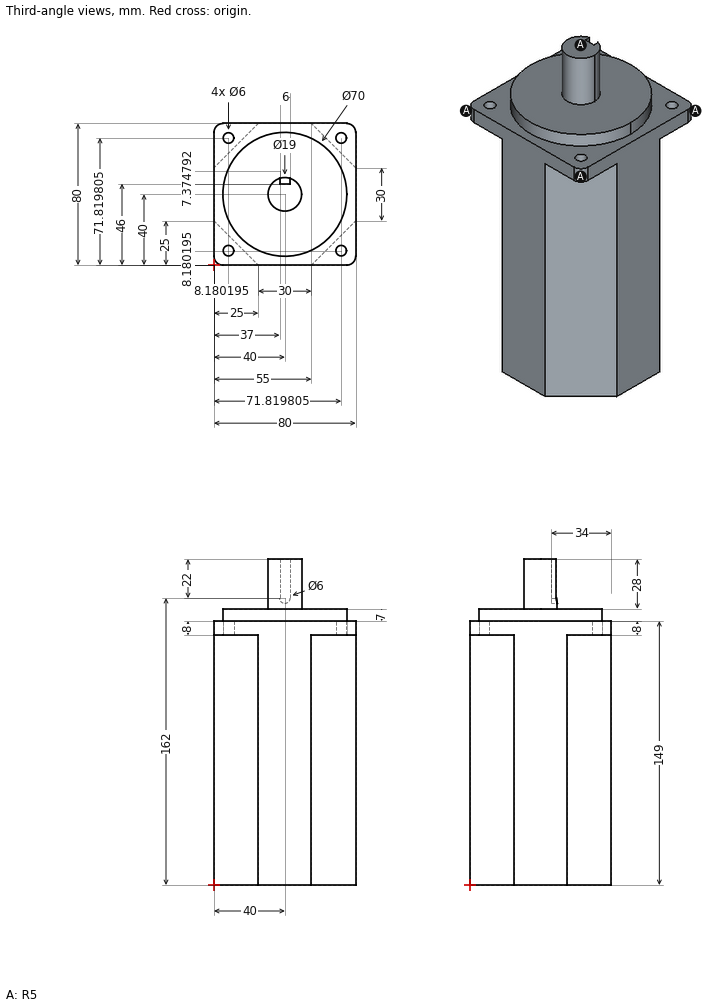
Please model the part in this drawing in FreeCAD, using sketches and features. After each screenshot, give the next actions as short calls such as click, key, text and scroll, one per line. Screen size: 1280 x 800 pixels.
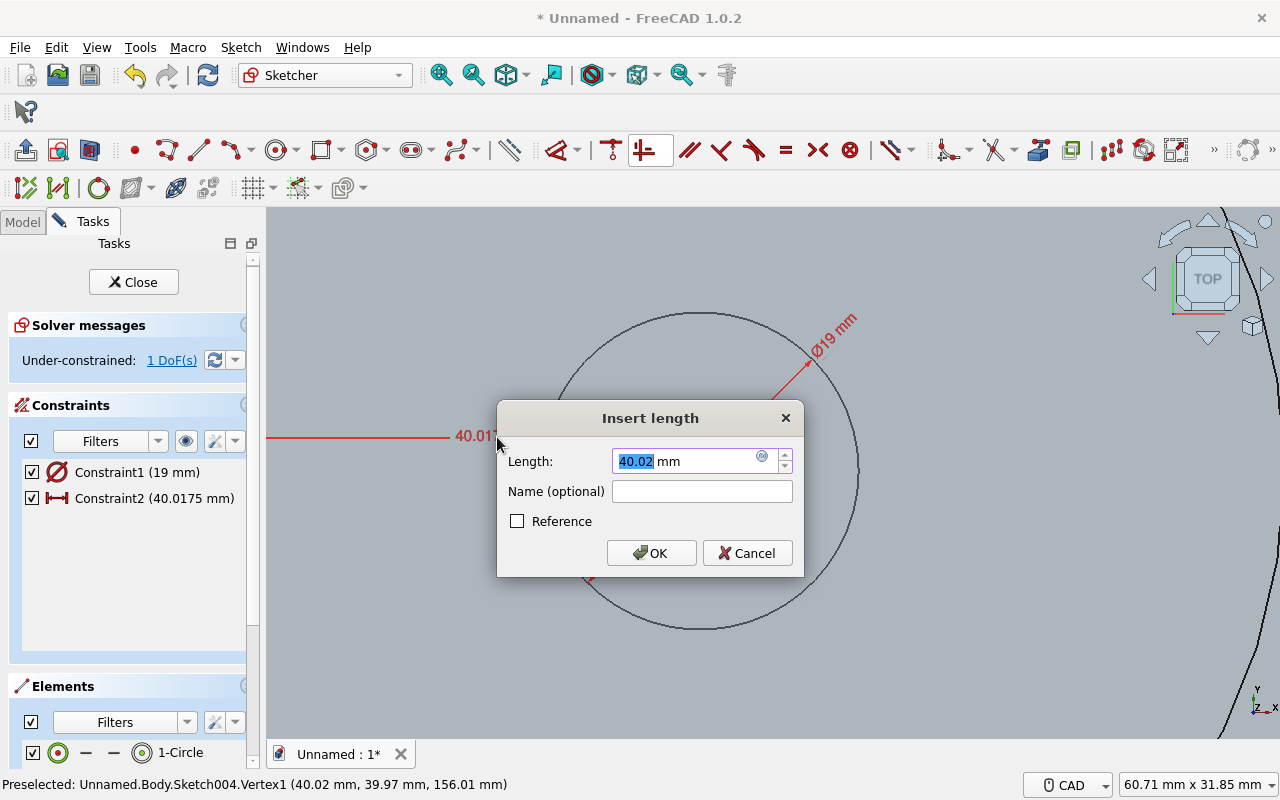
text(40)
key(Return)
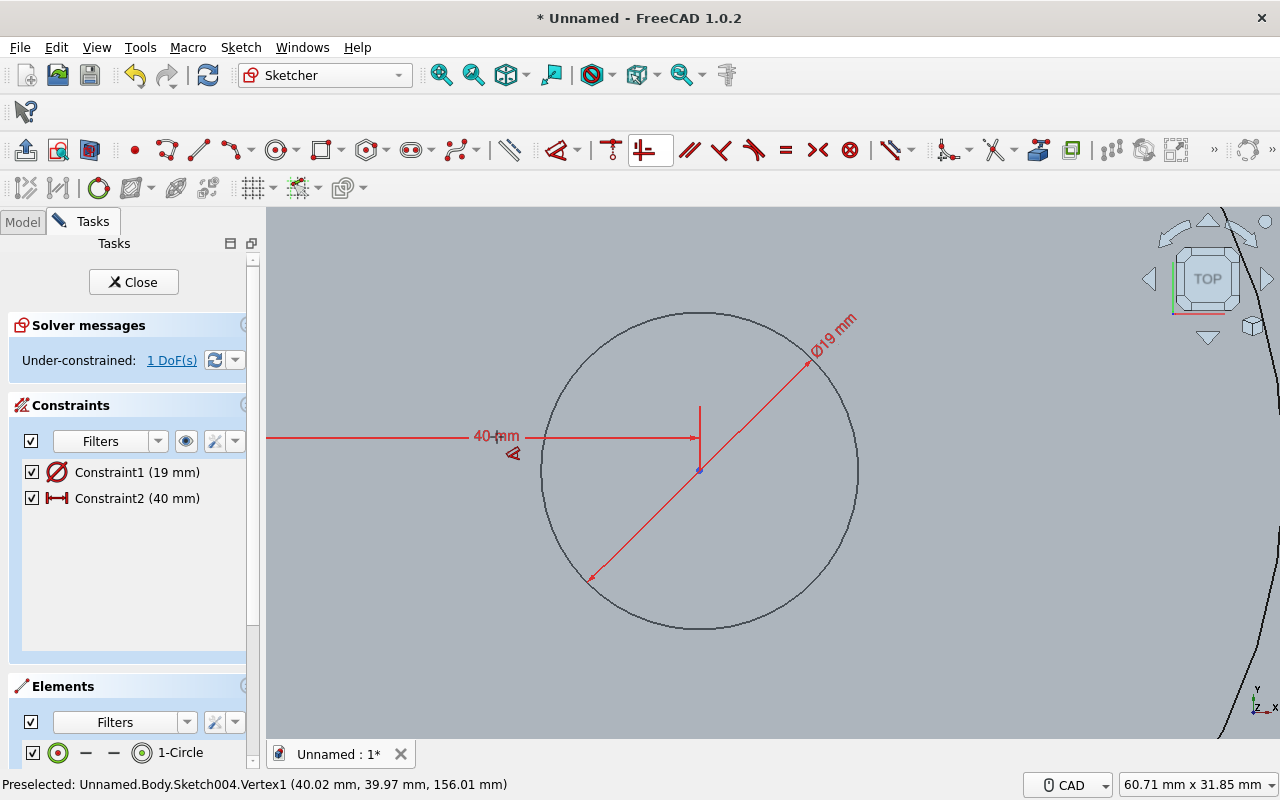
click(700, 471)
click(734, 591)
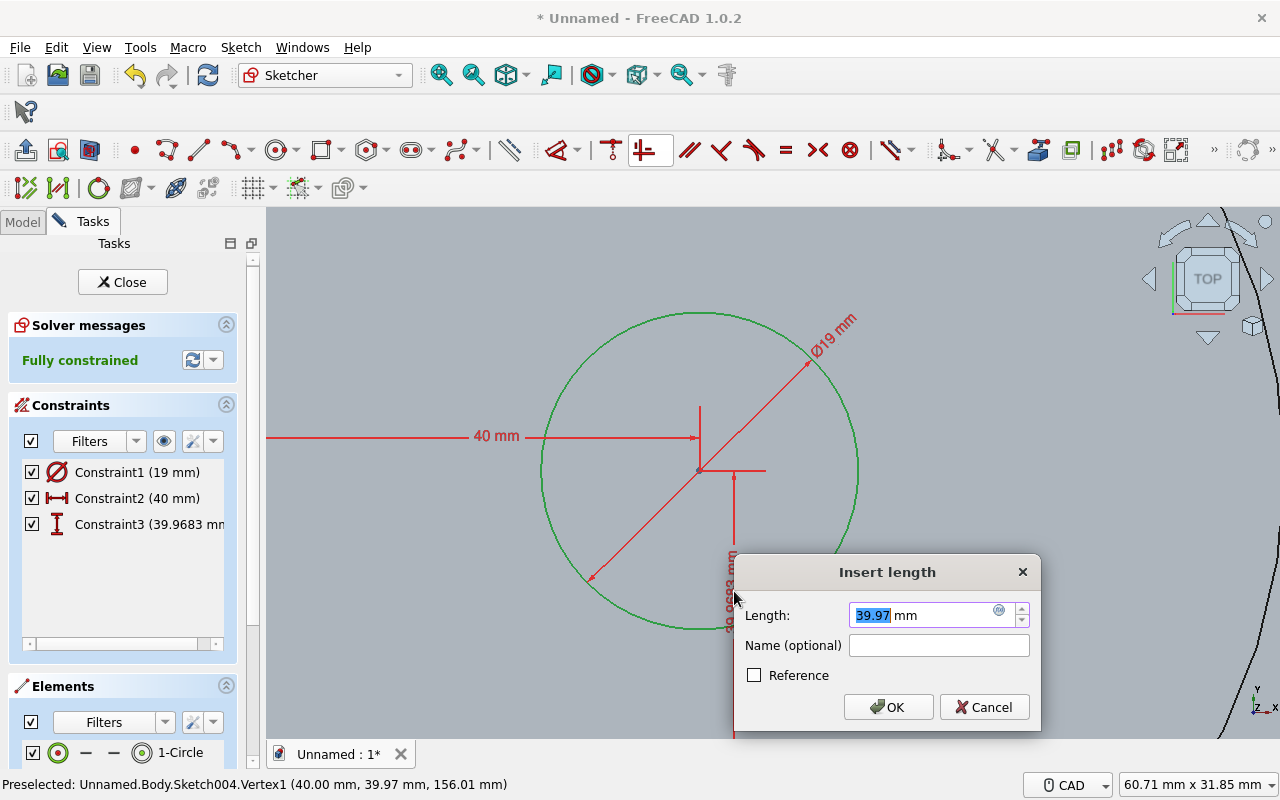
text(40)
key(Return)
key(Escape)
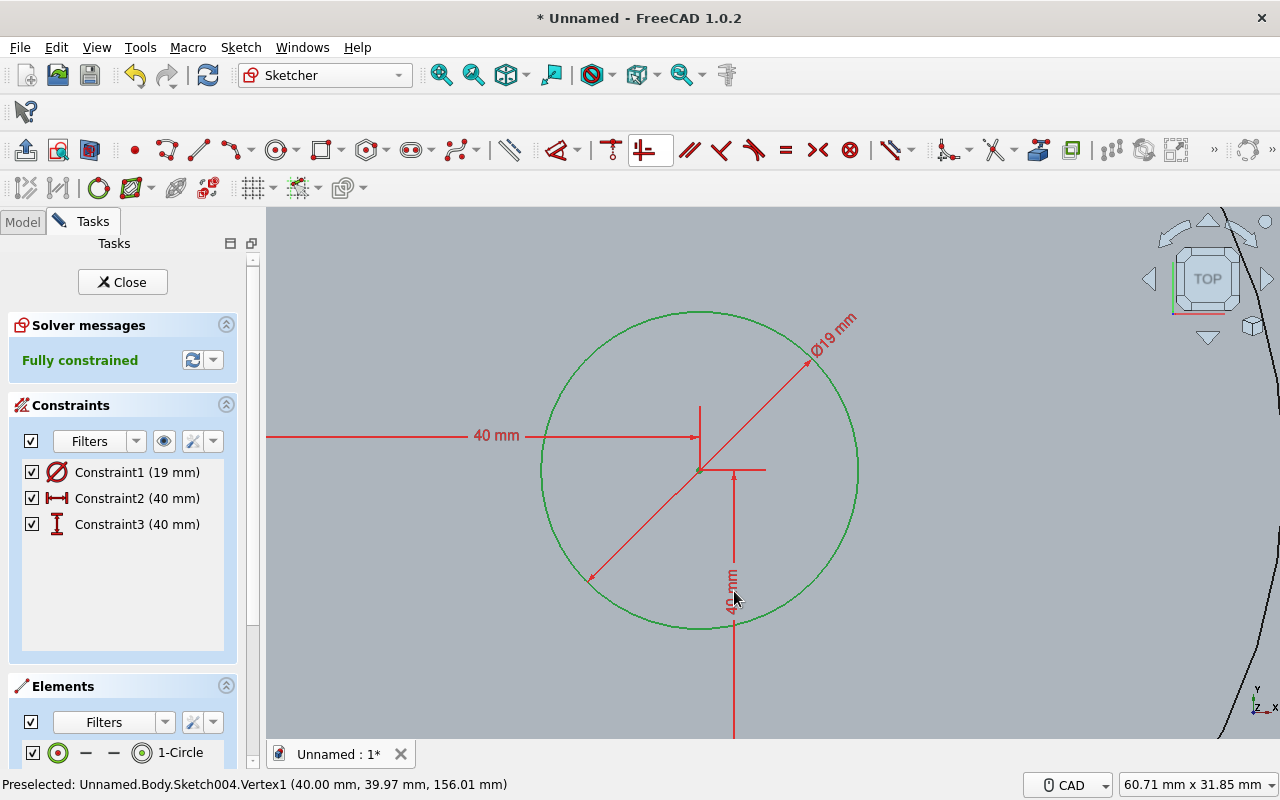
click(123, 282)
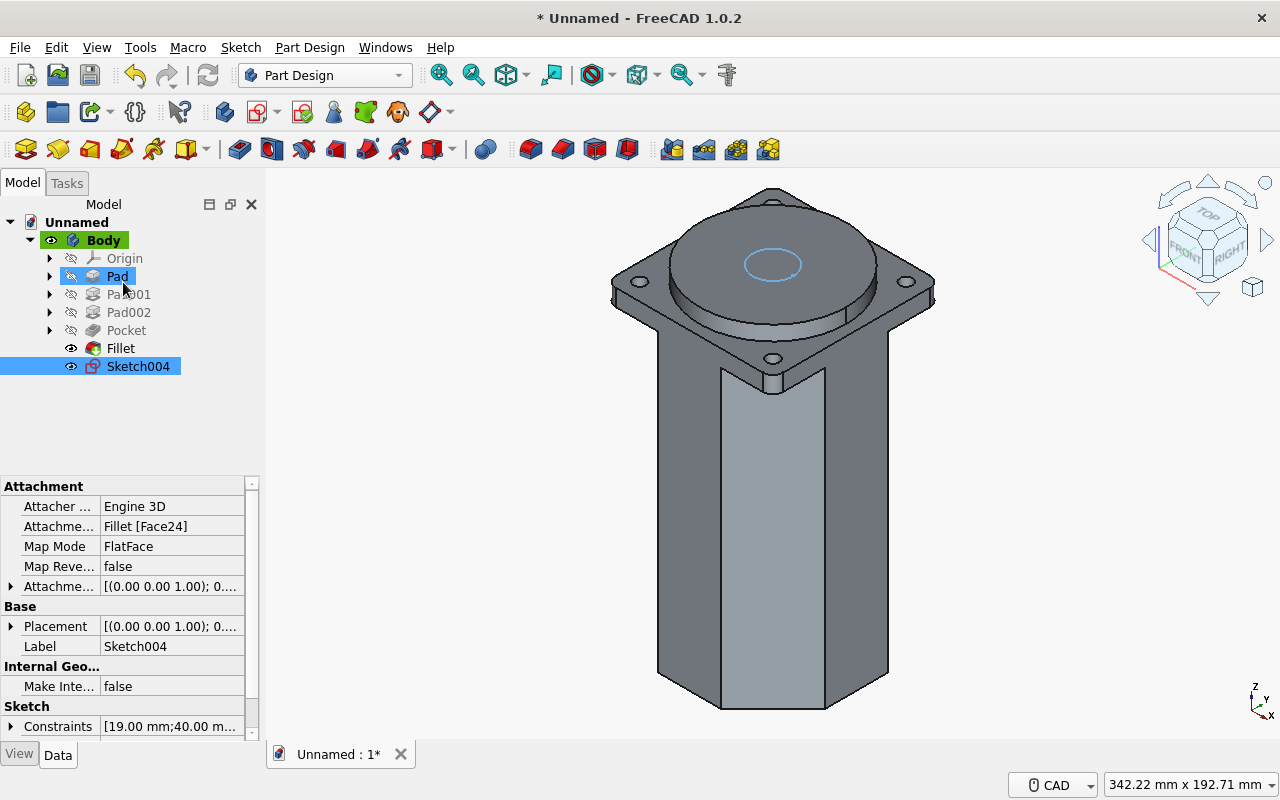
click(26, 150)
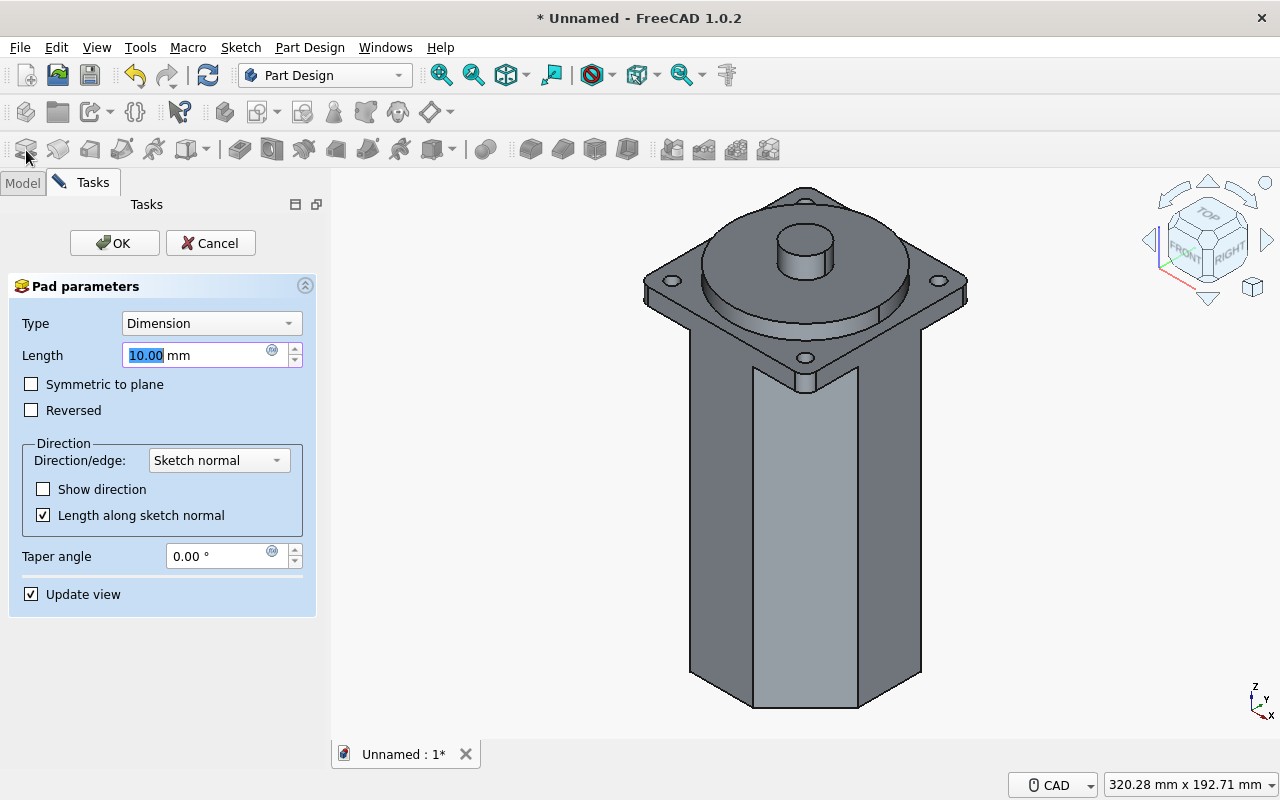
text(28)
key(Tab)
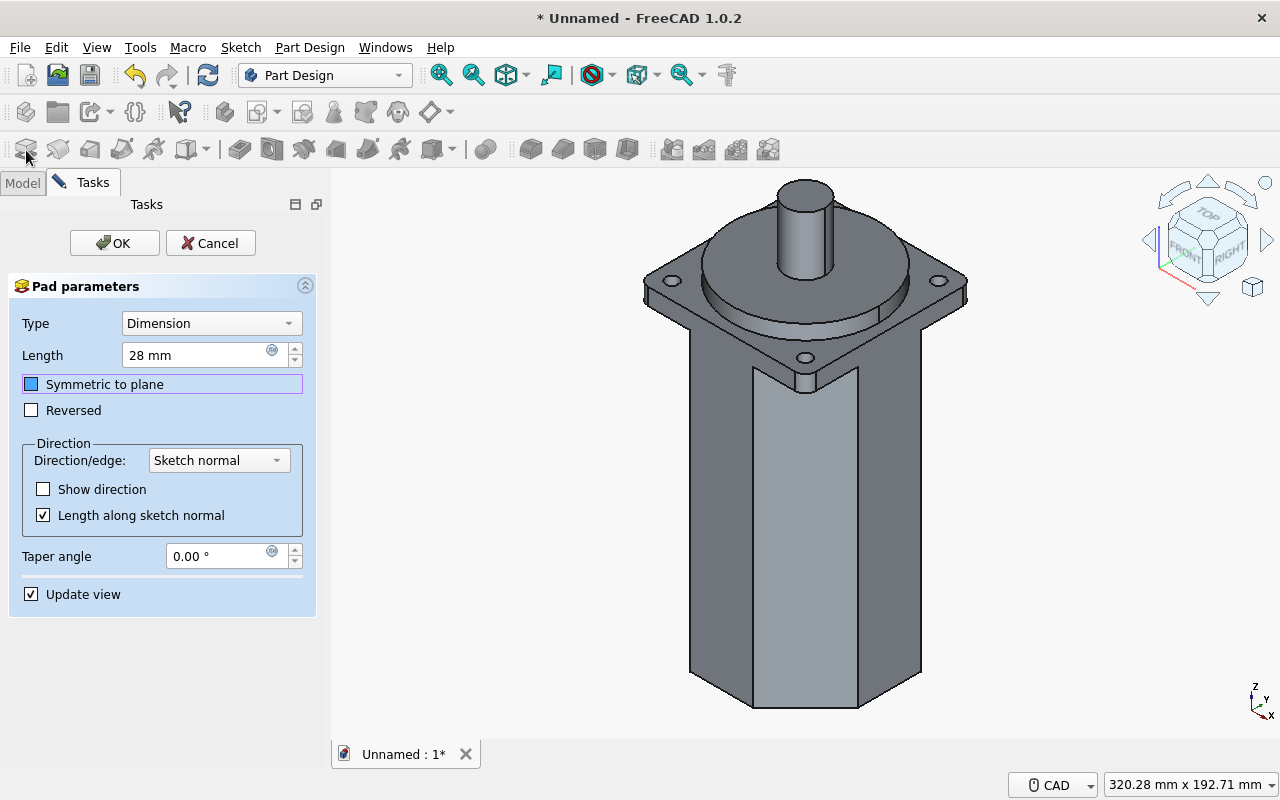
click(115, 243)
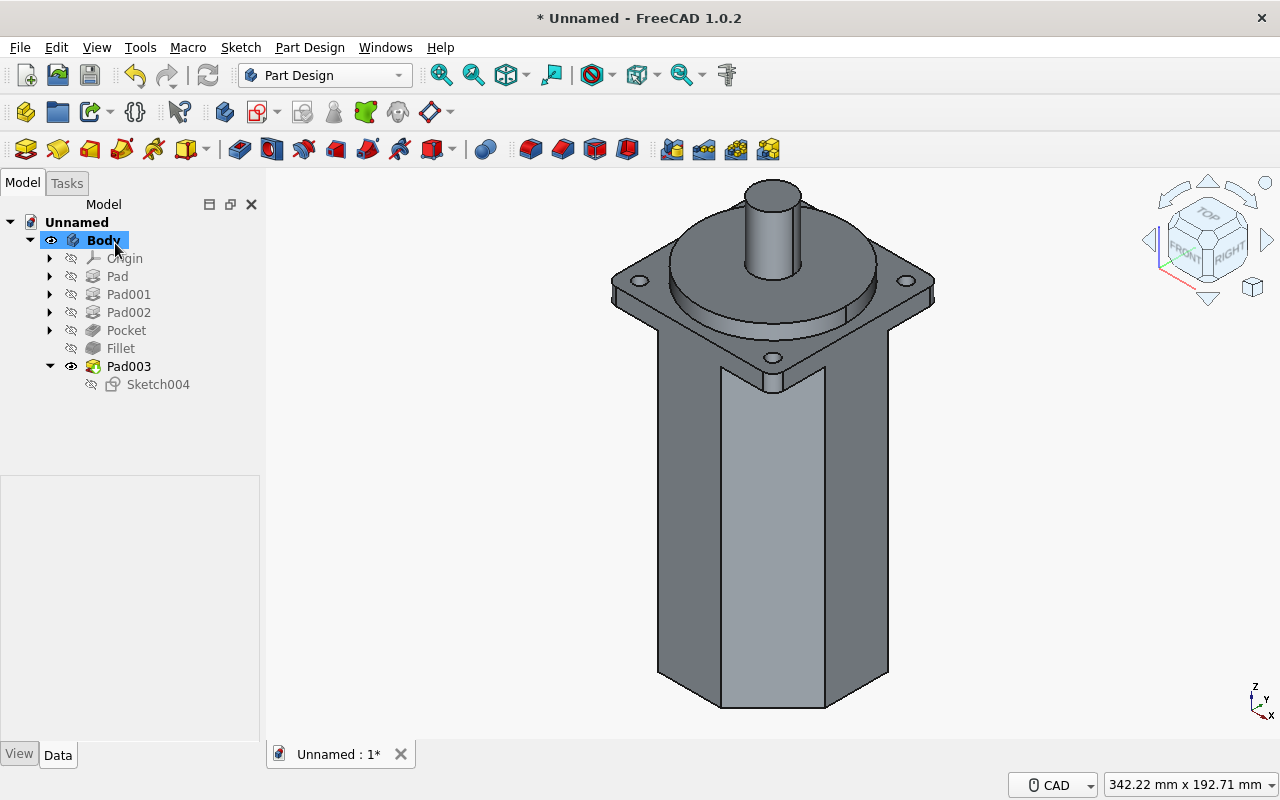
key(v)
key(f)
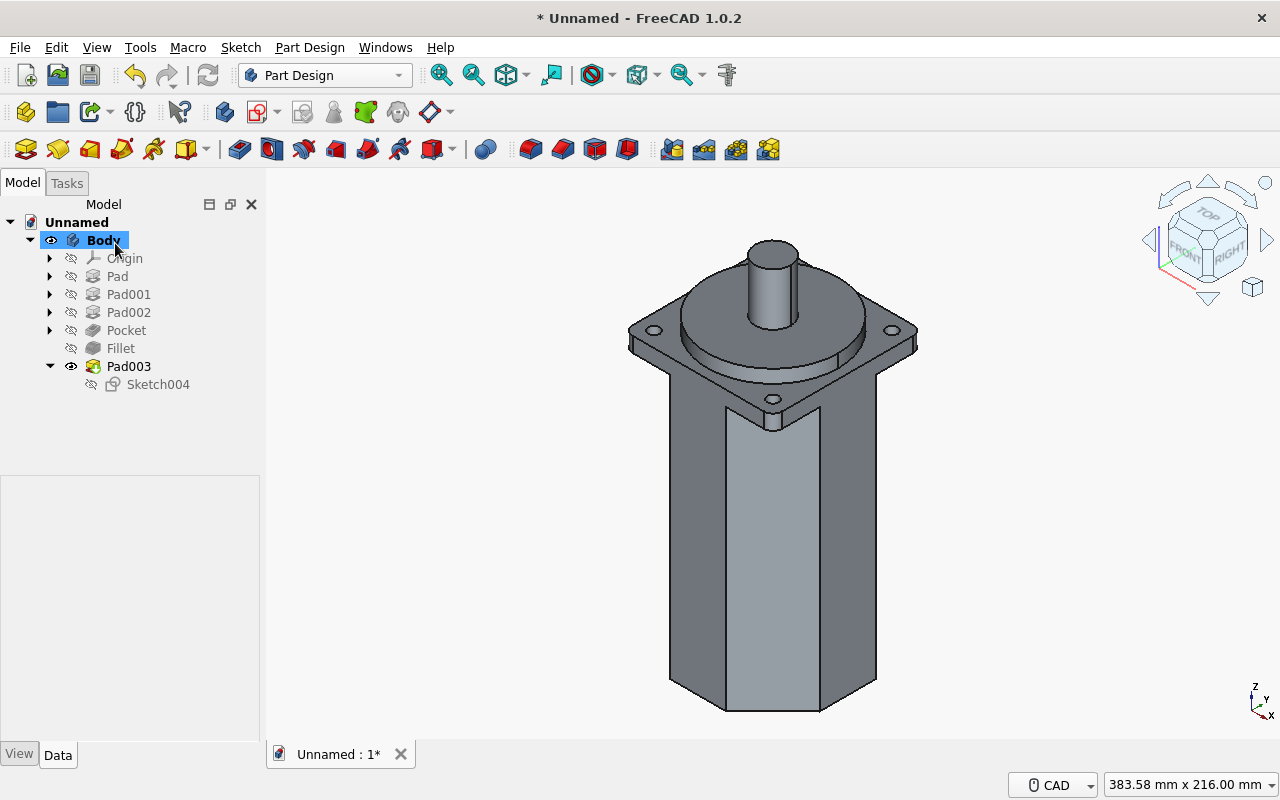
click(226, 112)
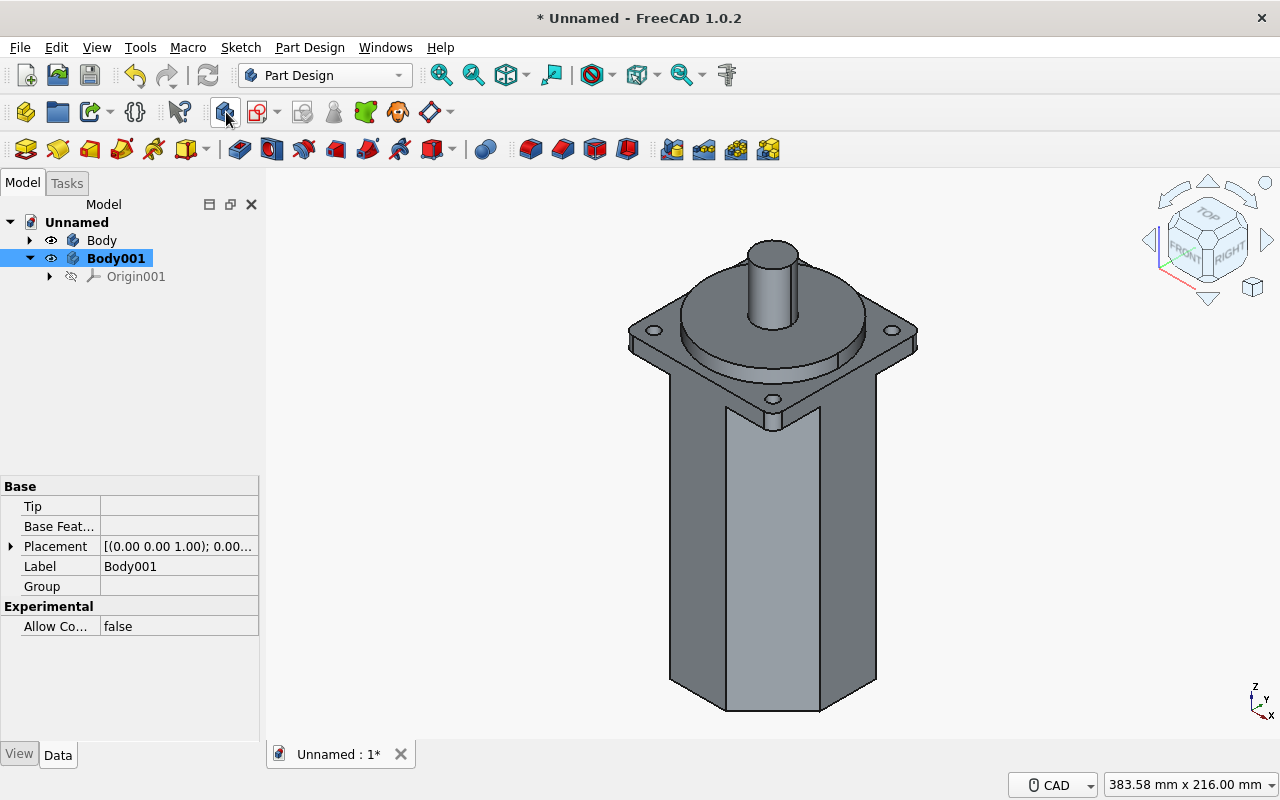
click(50, 276)